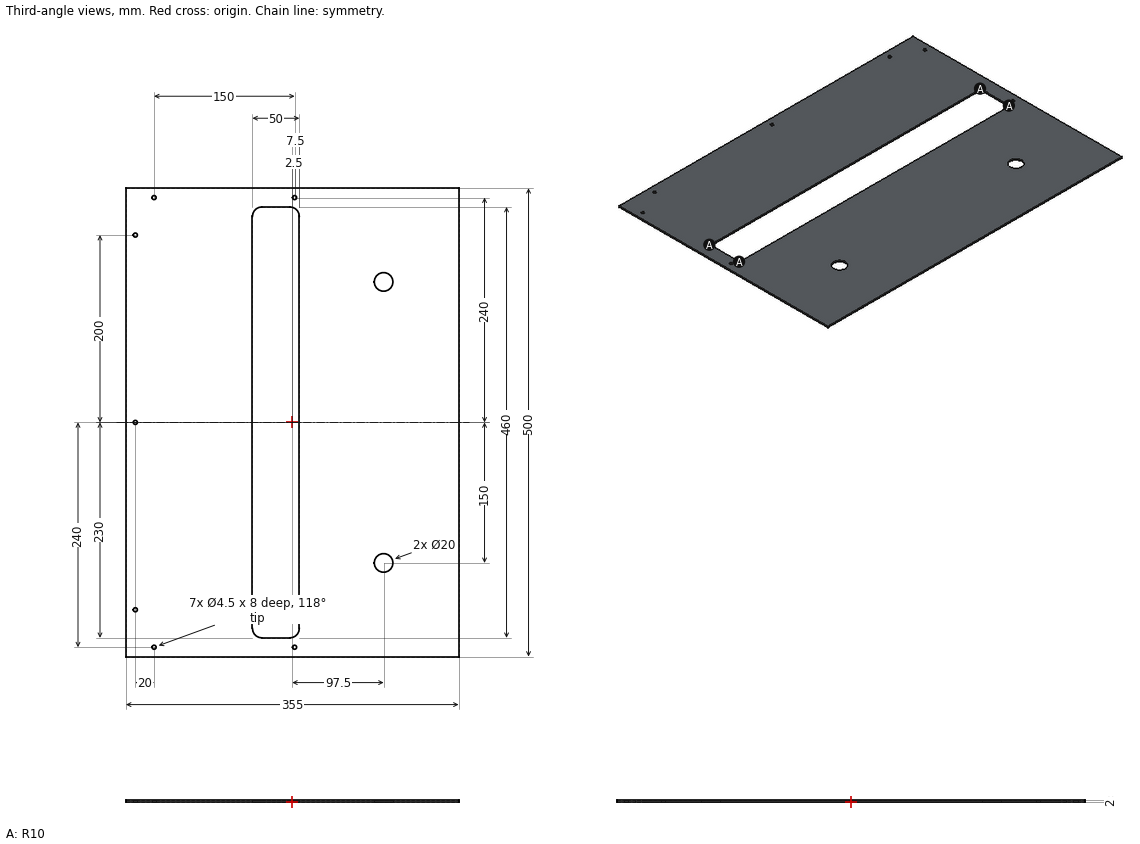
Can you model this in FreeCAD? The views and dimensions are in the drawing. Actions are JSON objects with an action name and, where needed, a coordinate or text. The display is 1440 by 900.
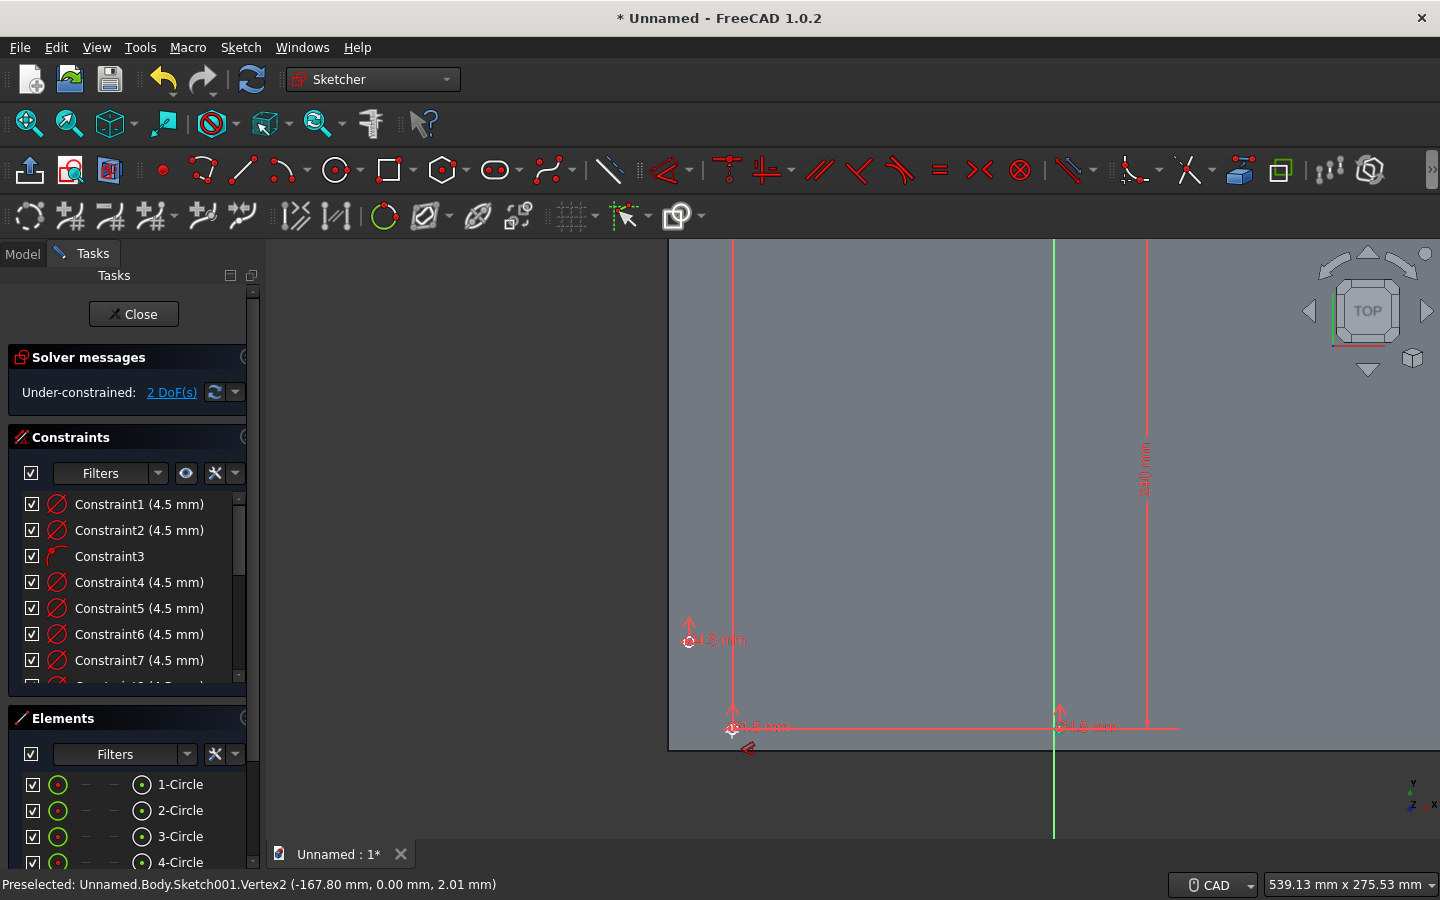
{"action": "left_click", "coordinate": [733, 729]}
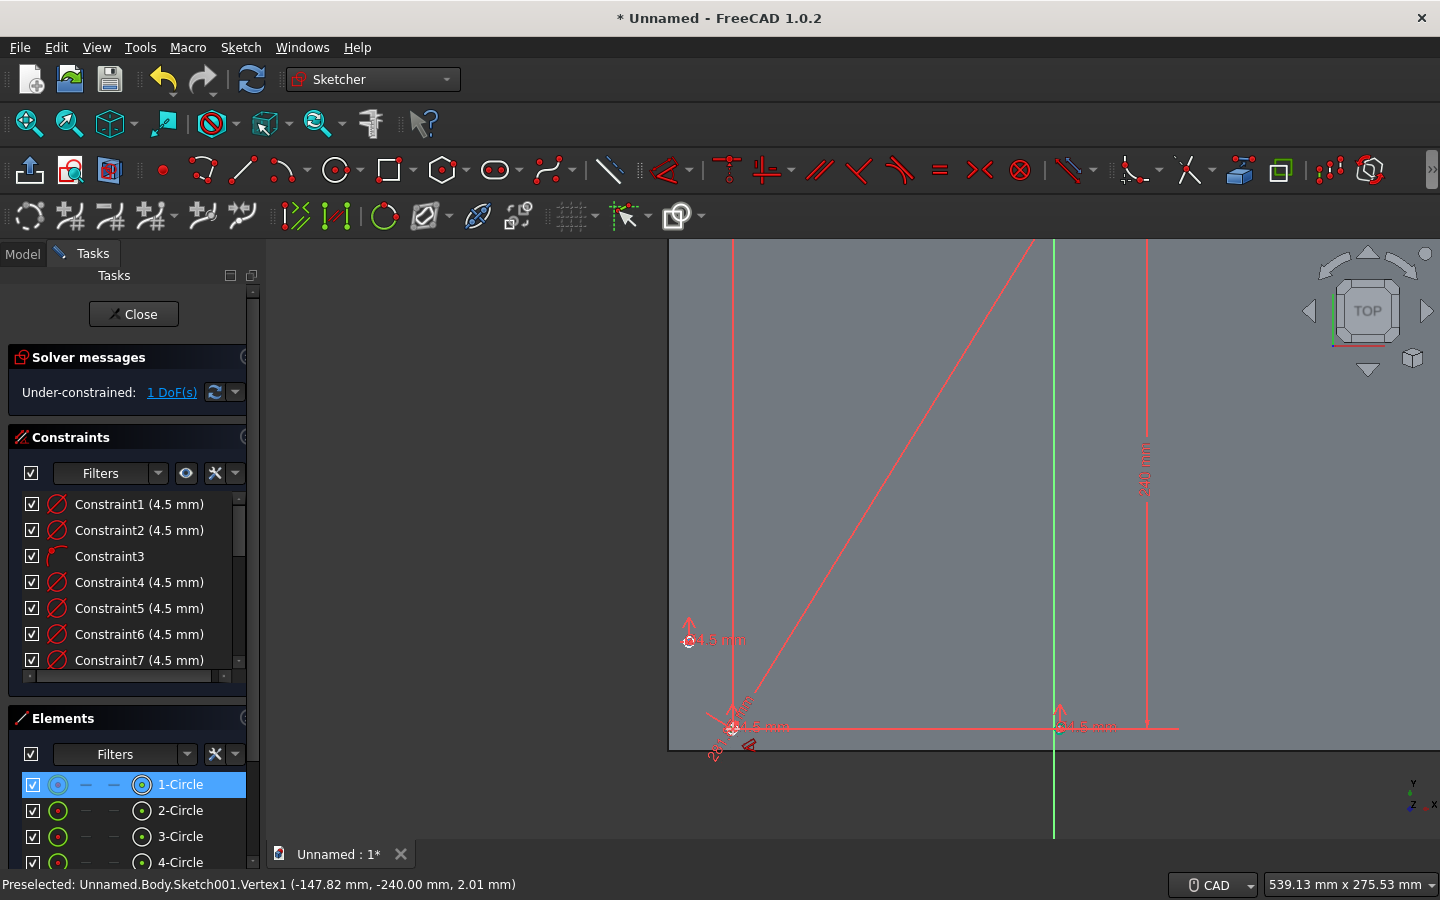
{"action": "scroll", "coordinate": [732, 732], "scroll_direction": "down", "scroll_amount": 5}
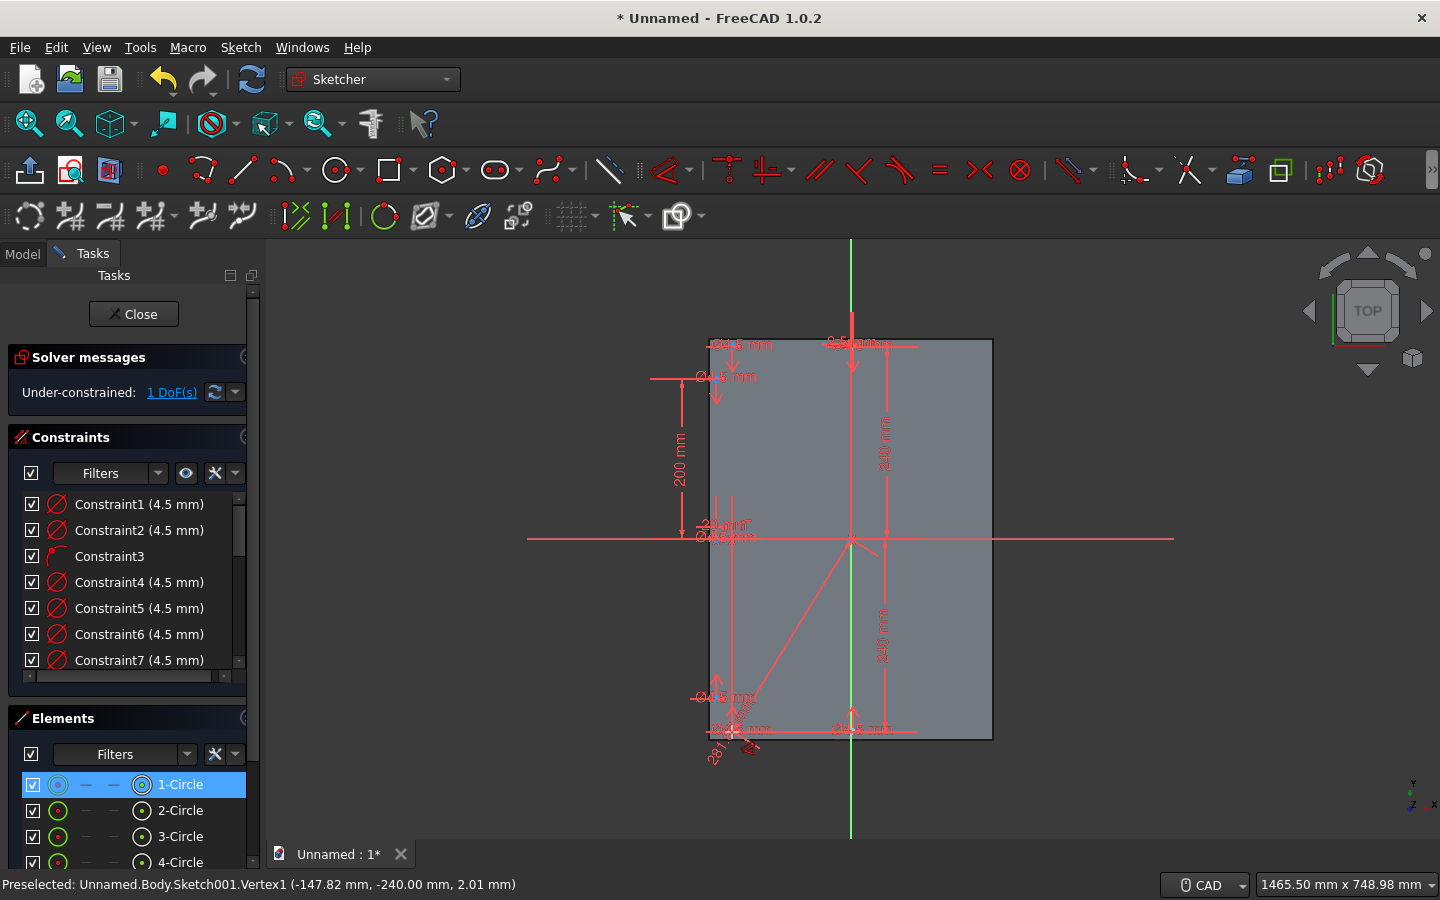
{"action": "scroll", "coordinate": [716, 379], "scroll_direction": "up", "scroll_amount": 5}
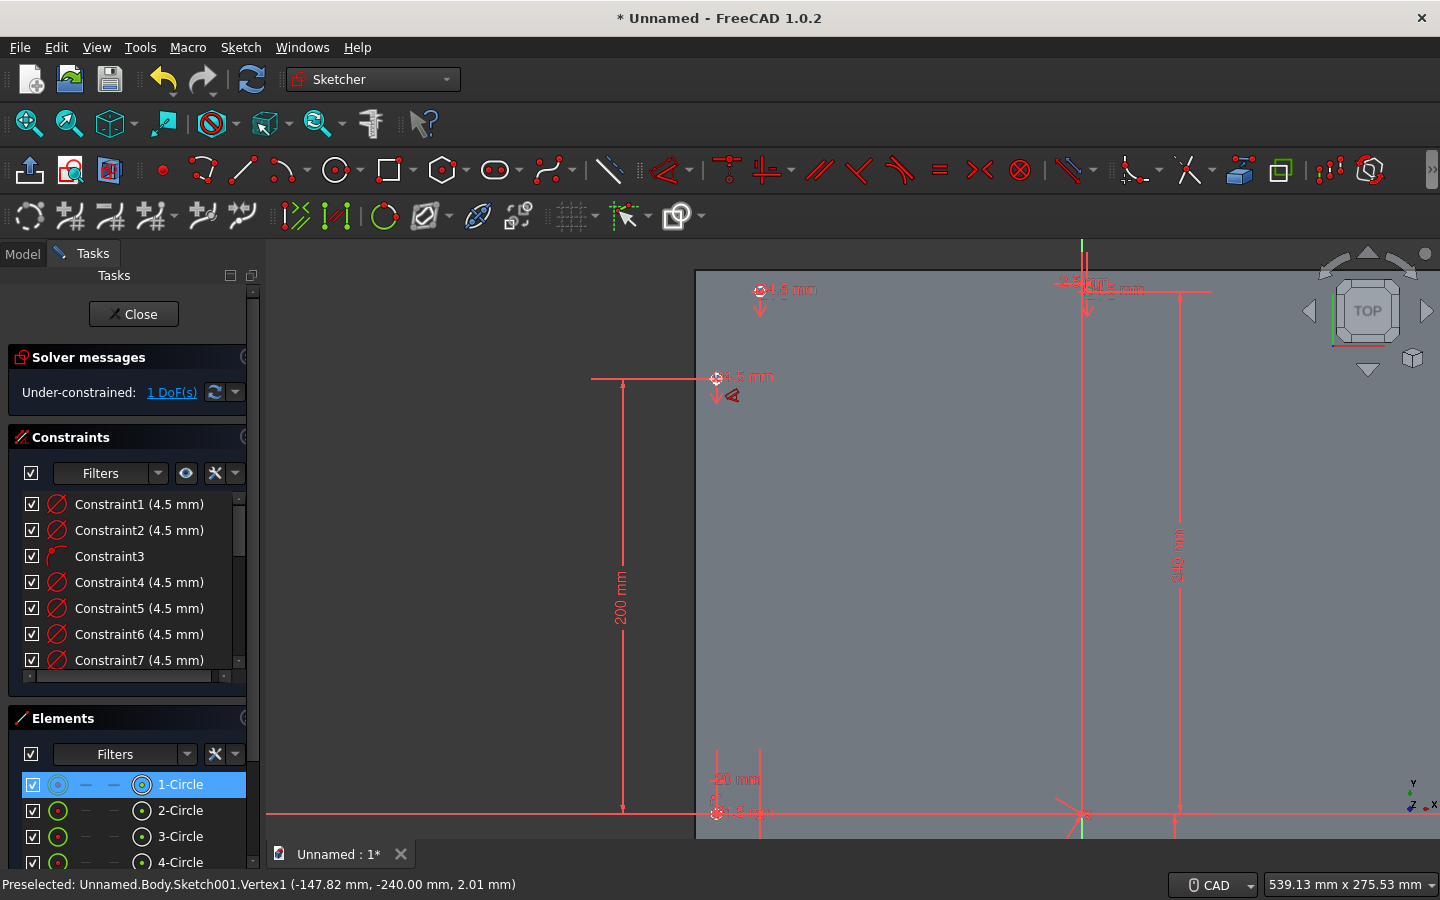
{"action": "left_click", "coordinate": [717, 379]}
{"action": "left_click", "coordinate": [738, 345]}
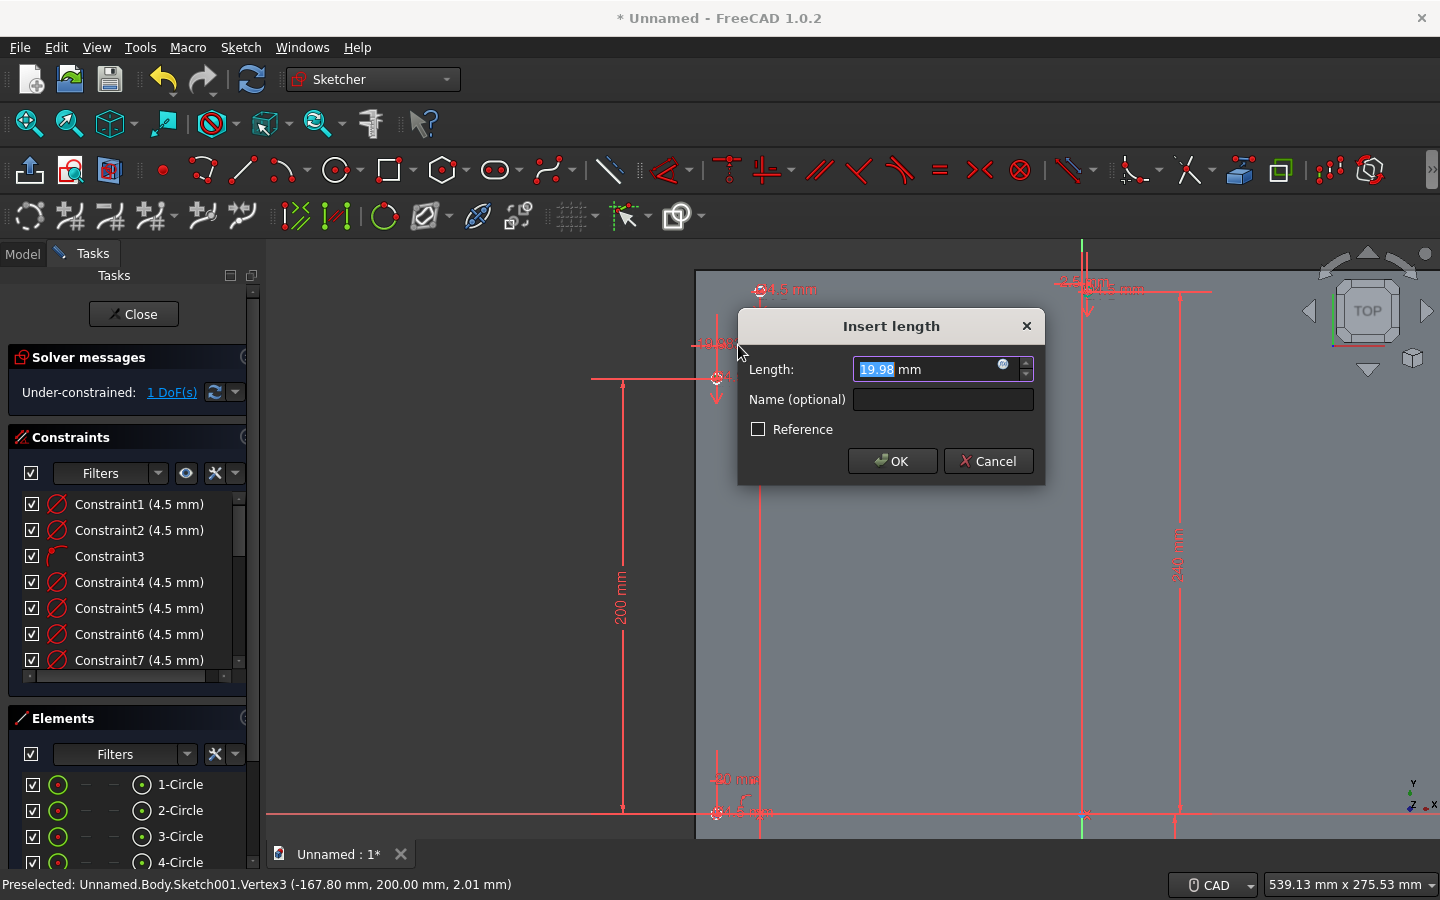
{"action": "type", "text": "20"}
{"action": "key", "text": "Return"}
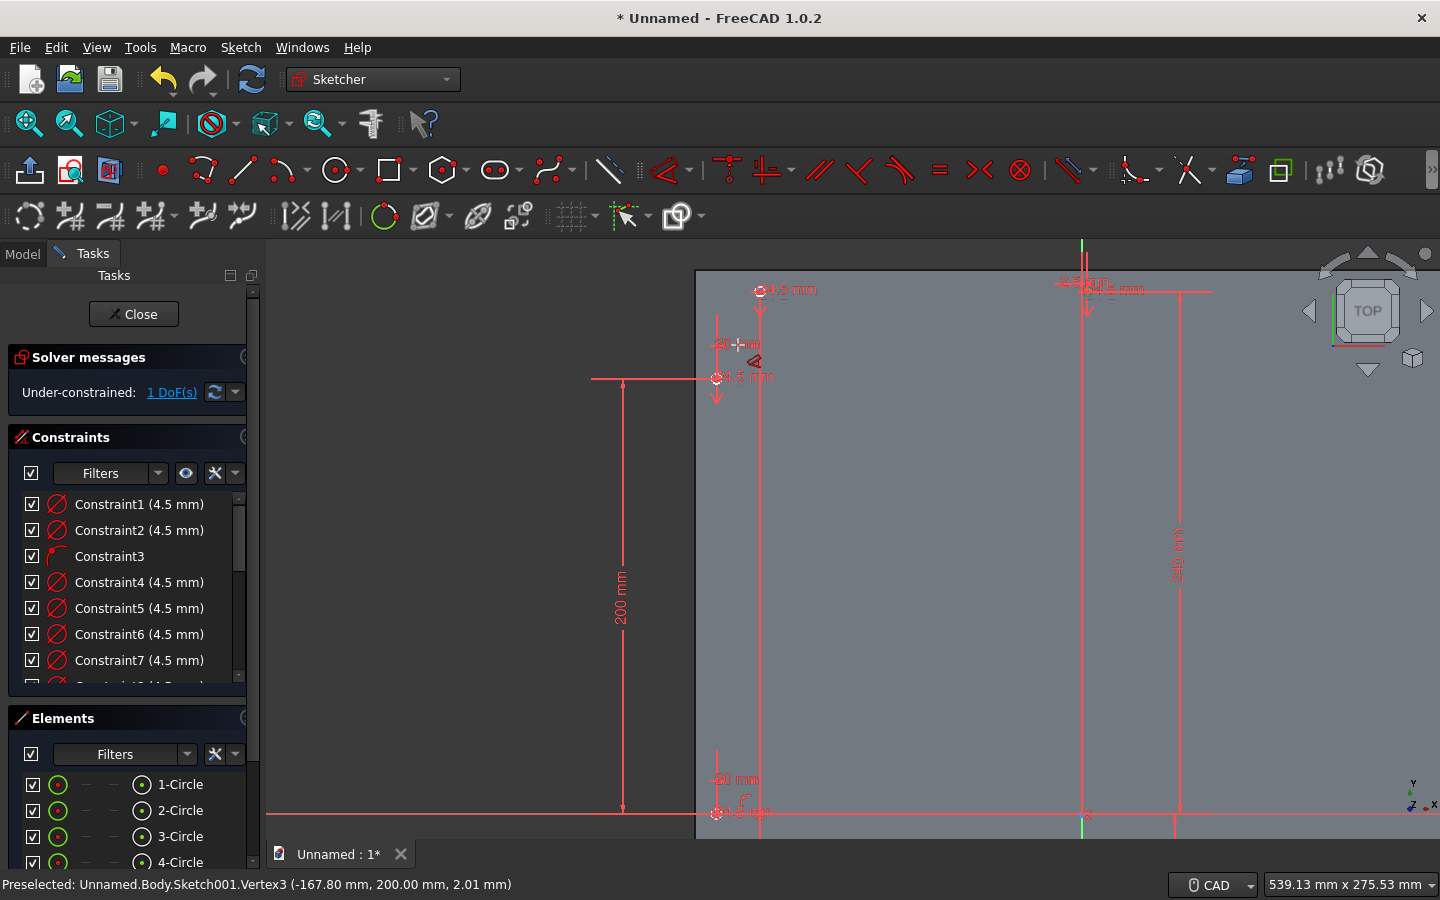
{"action": "left_click", "coordinate": [760, 292]}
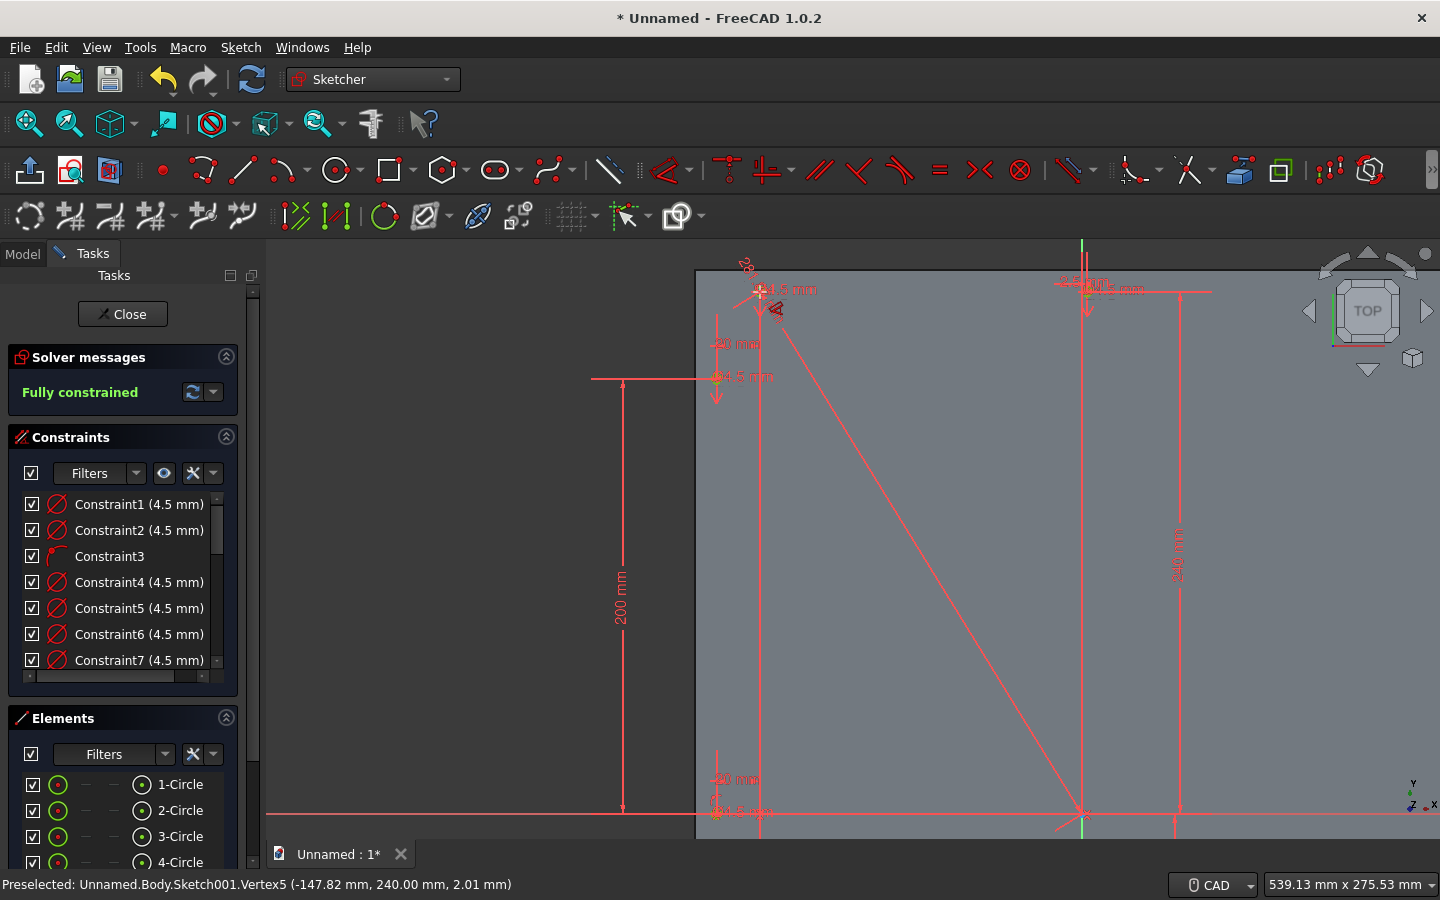
{"action": "left_click", "coordinate": [1087, 292]}
{"action": "left_click", "coordinate": [924, 326]}